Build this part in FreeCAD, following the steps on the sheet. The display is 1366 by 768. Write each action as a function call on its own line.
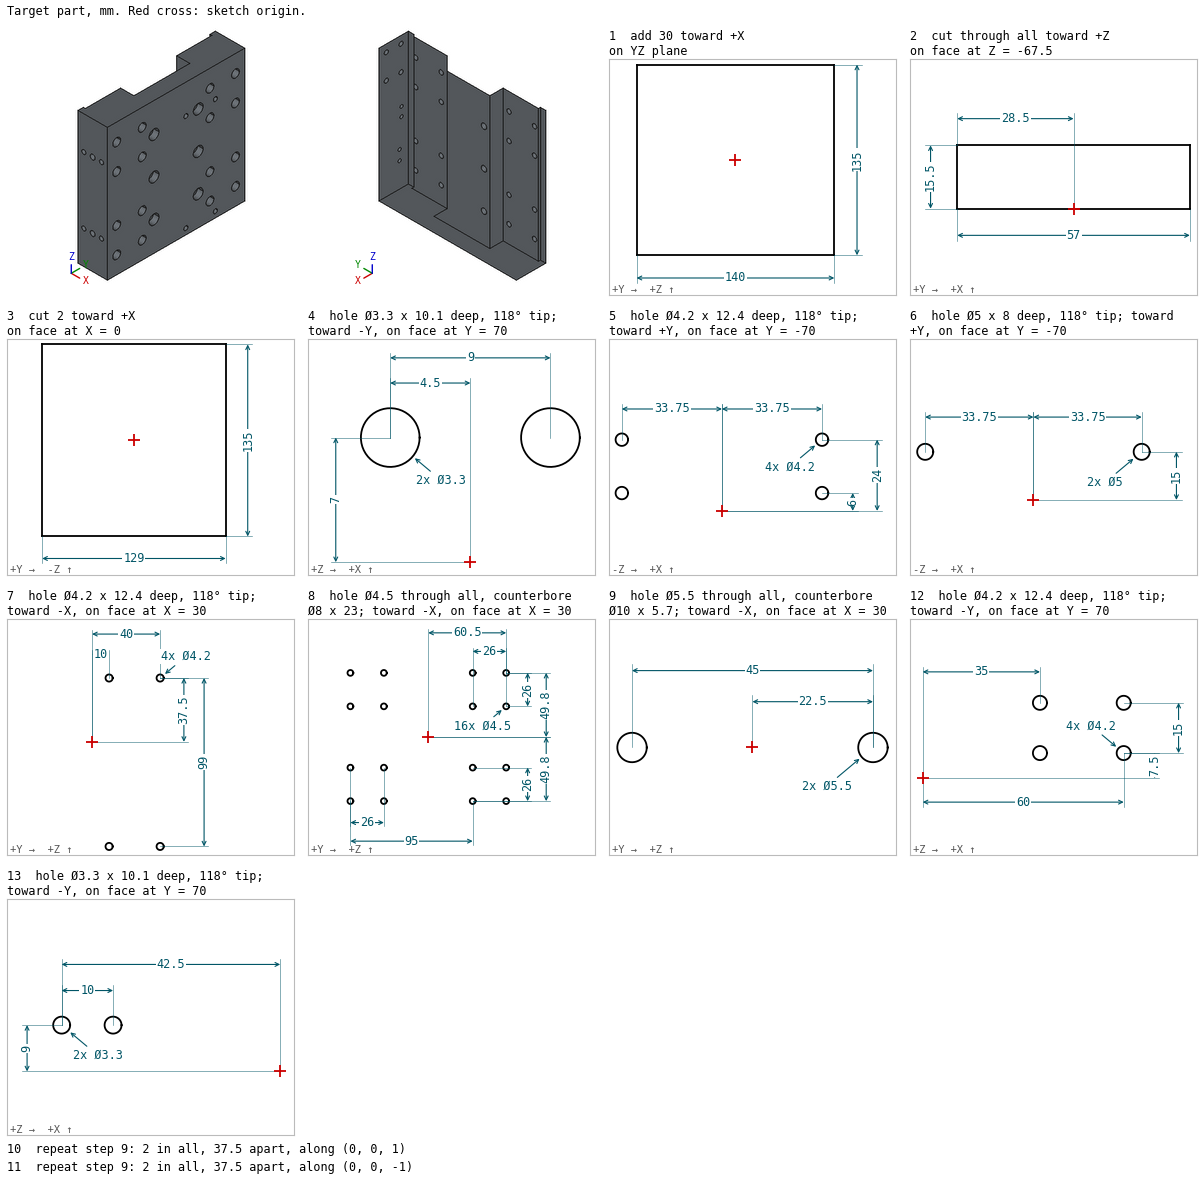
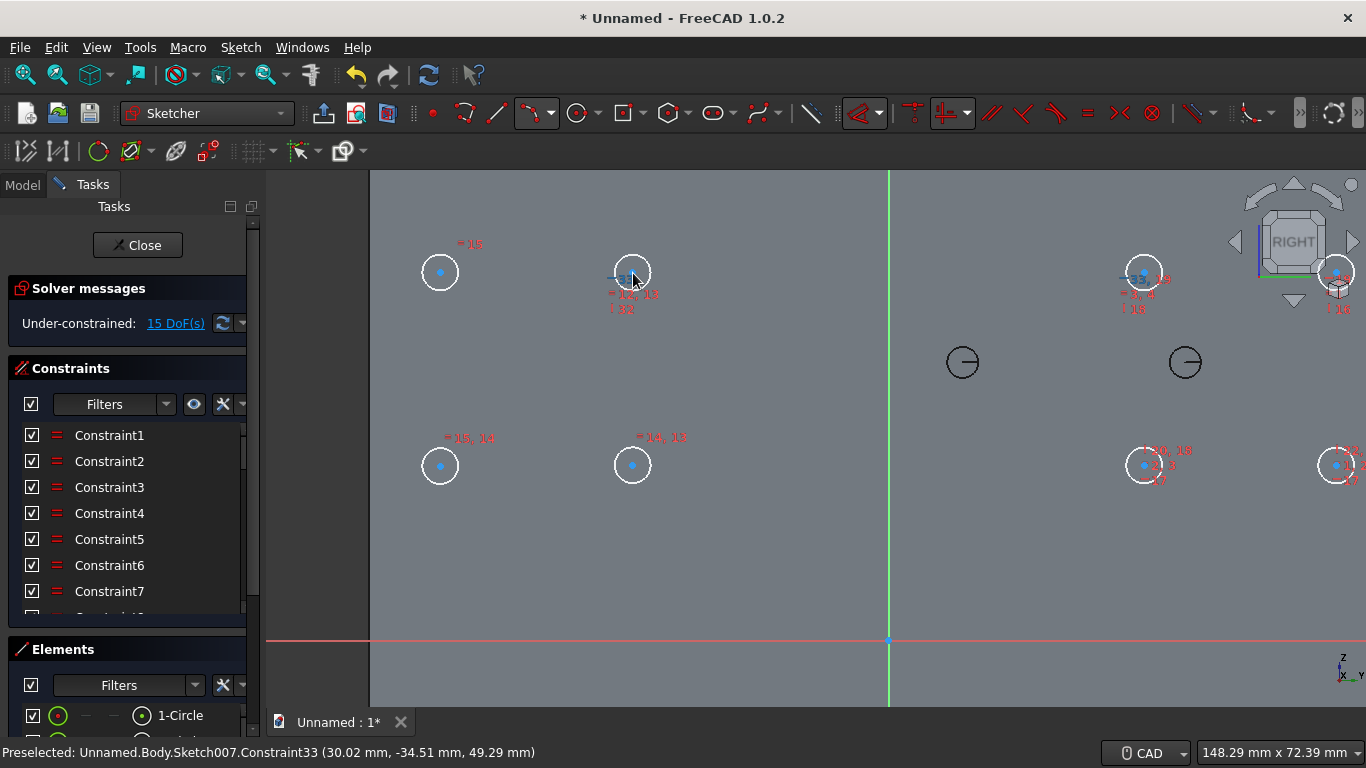
scroll(633, 273, up, 4)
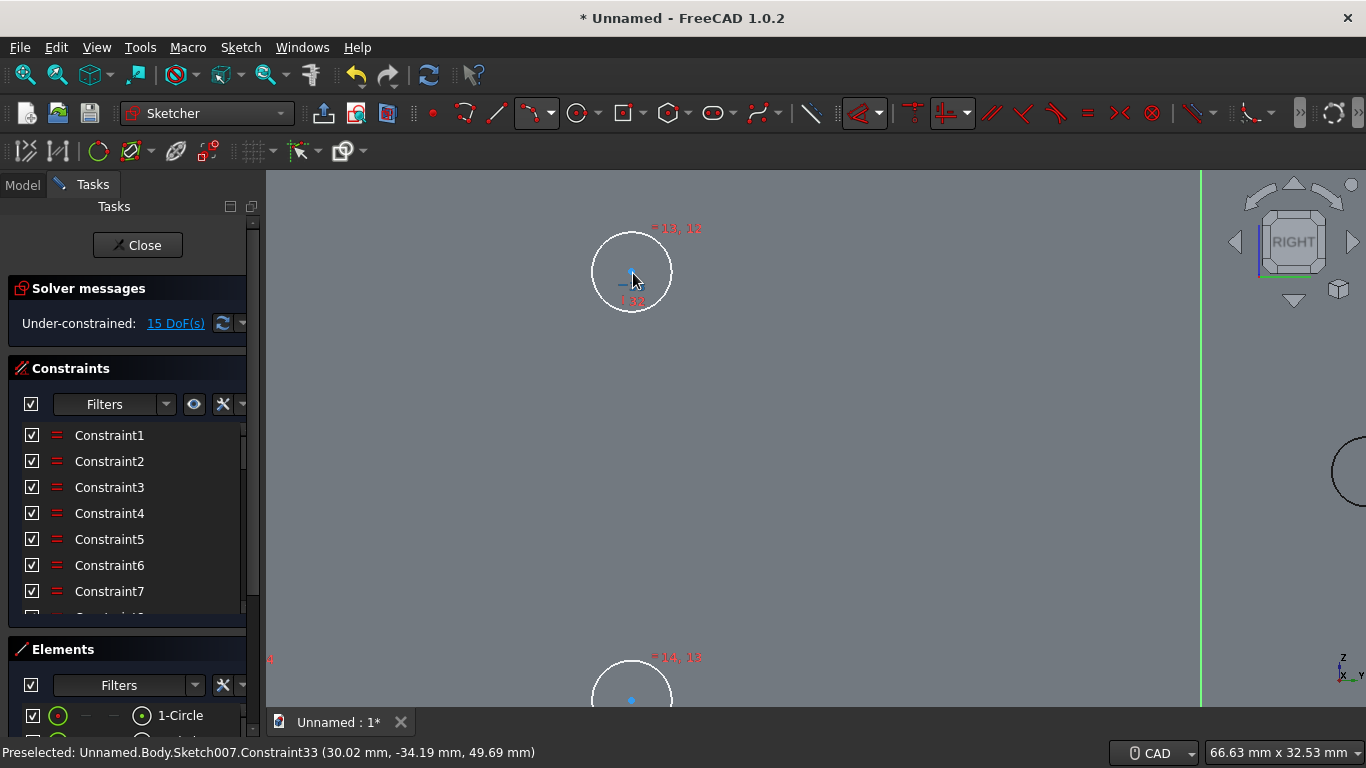
click(632, 272)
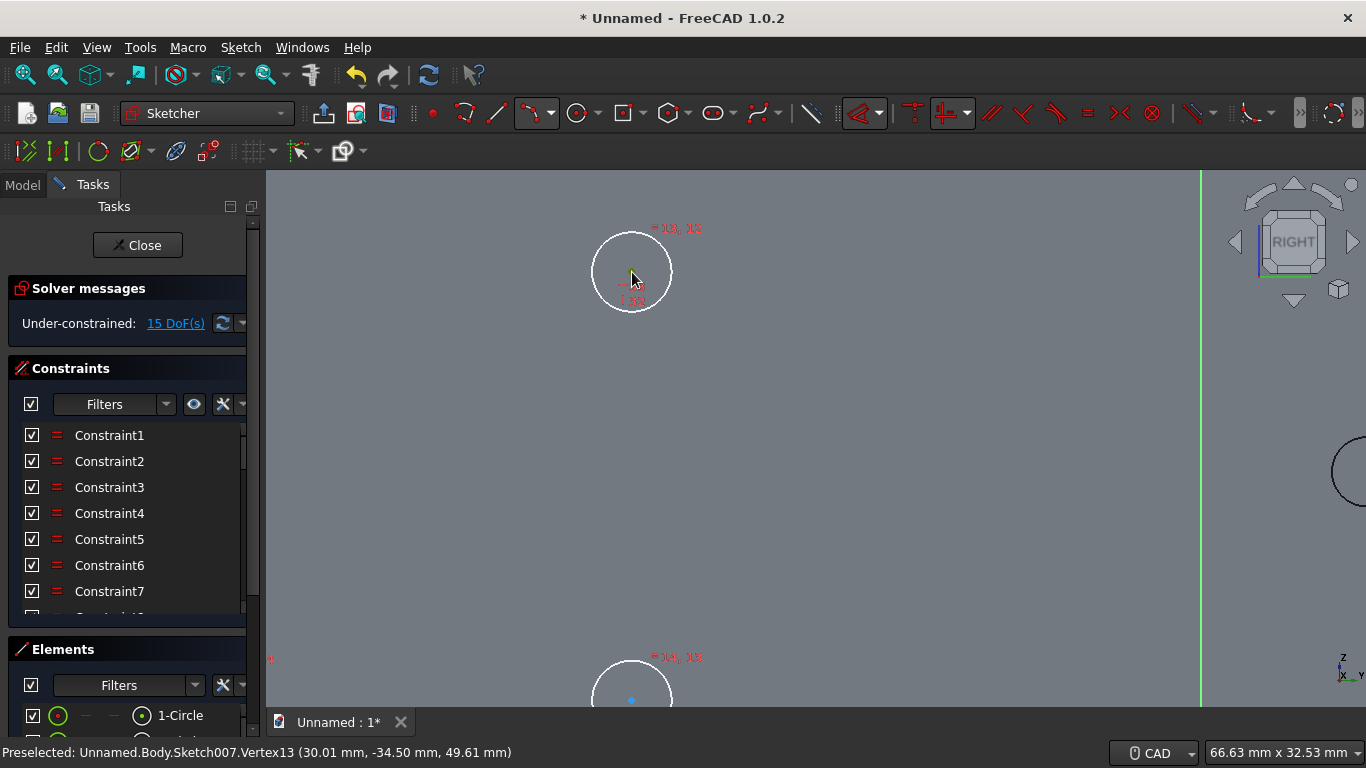
scroll(633, 273, down, 8)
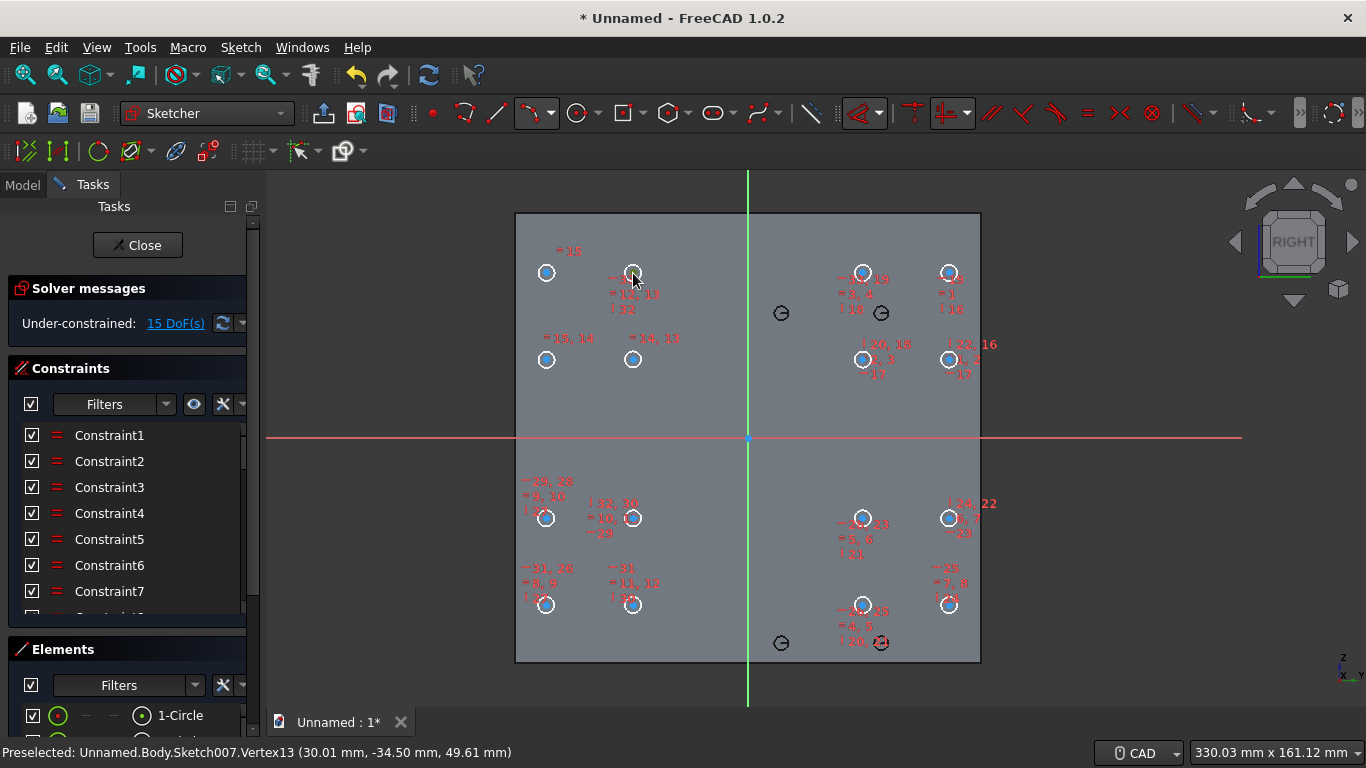
click(633, 359)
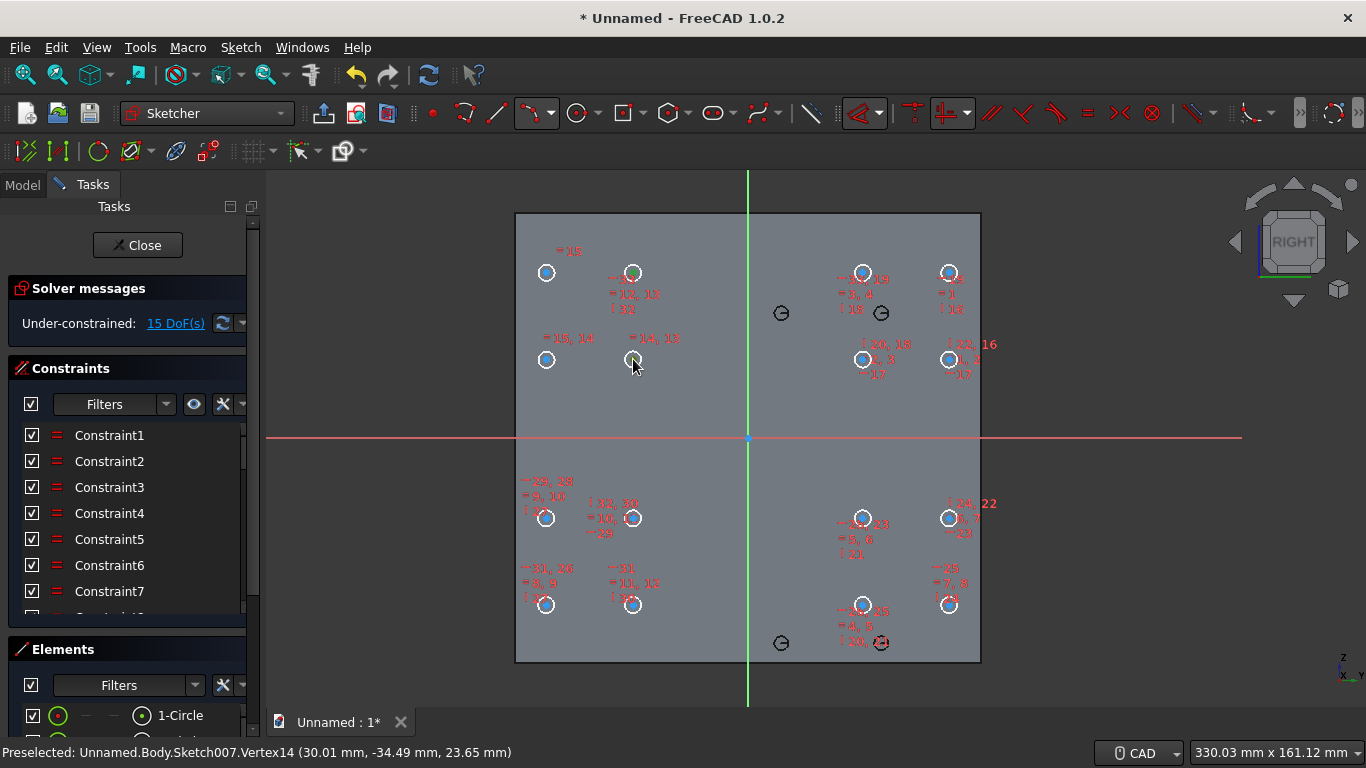
key(v)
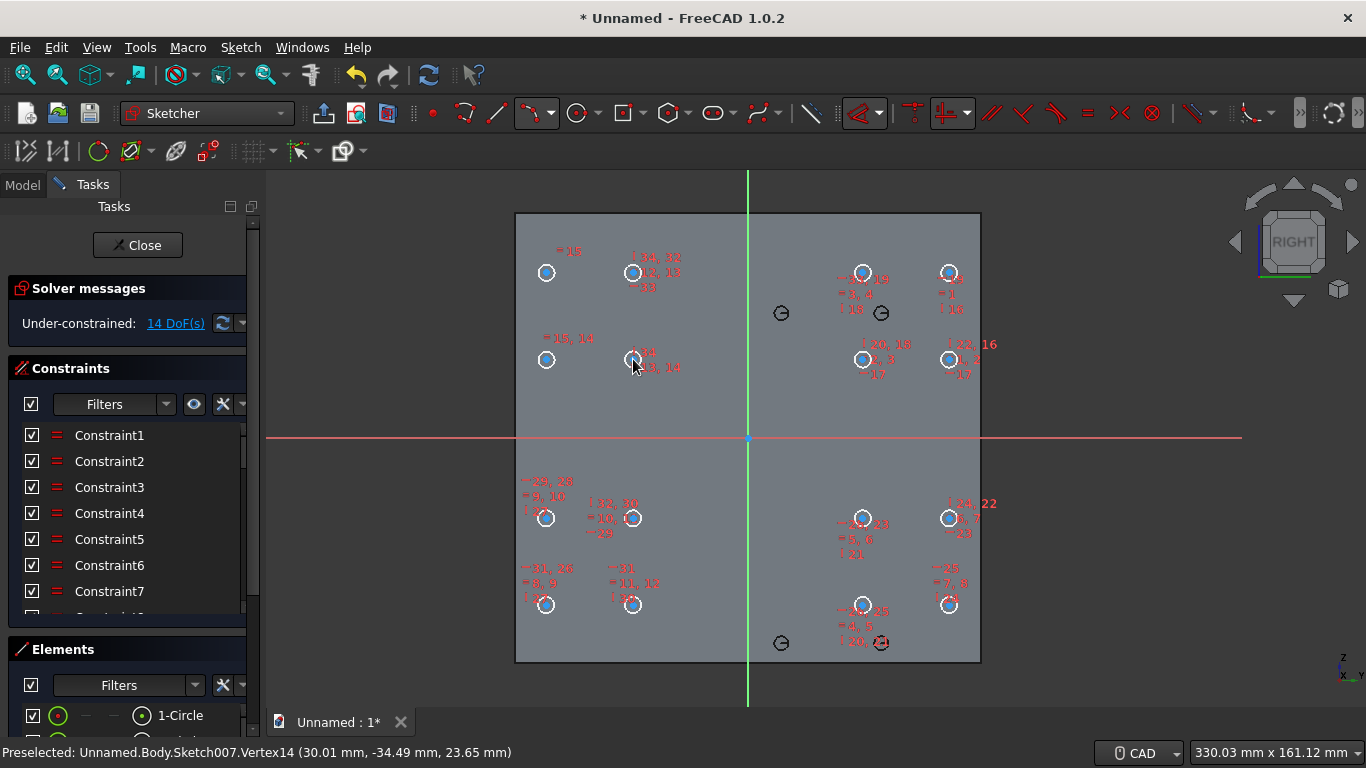
click(863, 360)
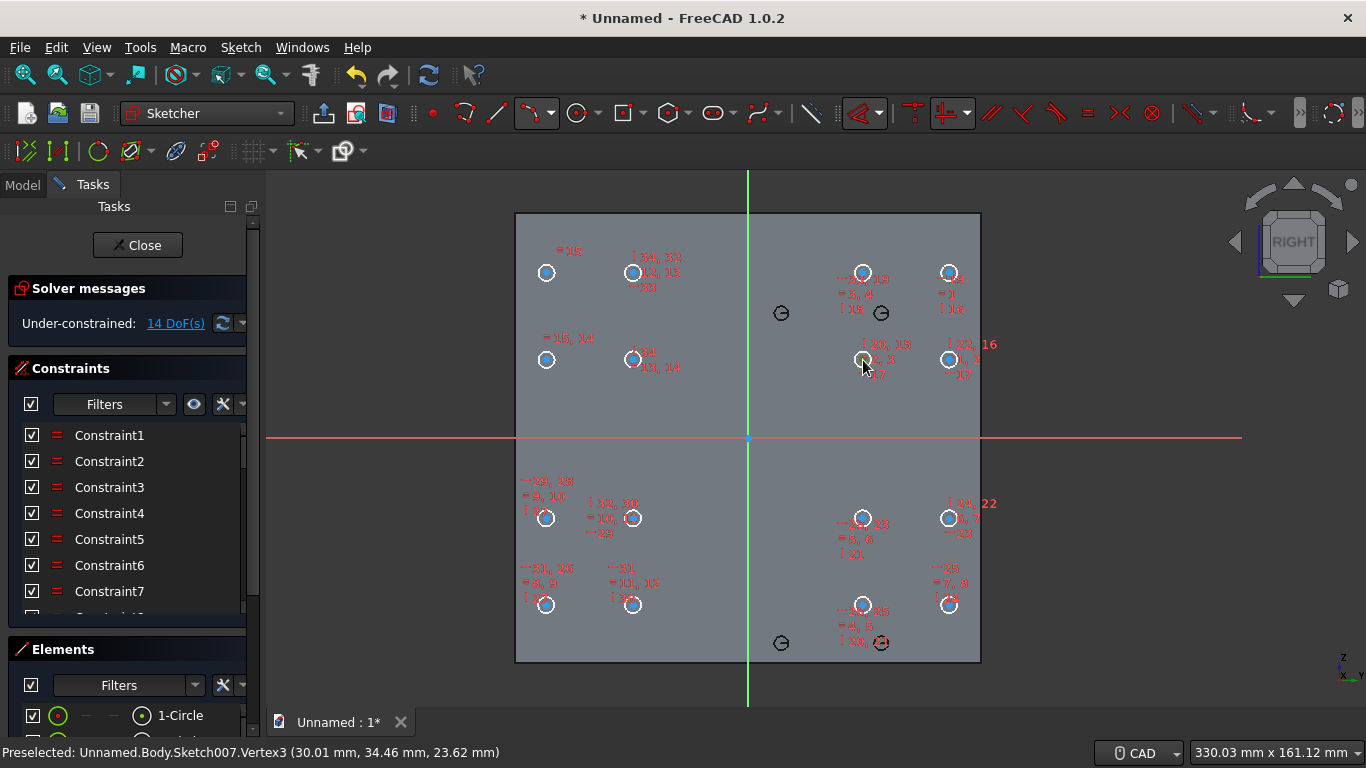
scroll(633, 359, up, 4)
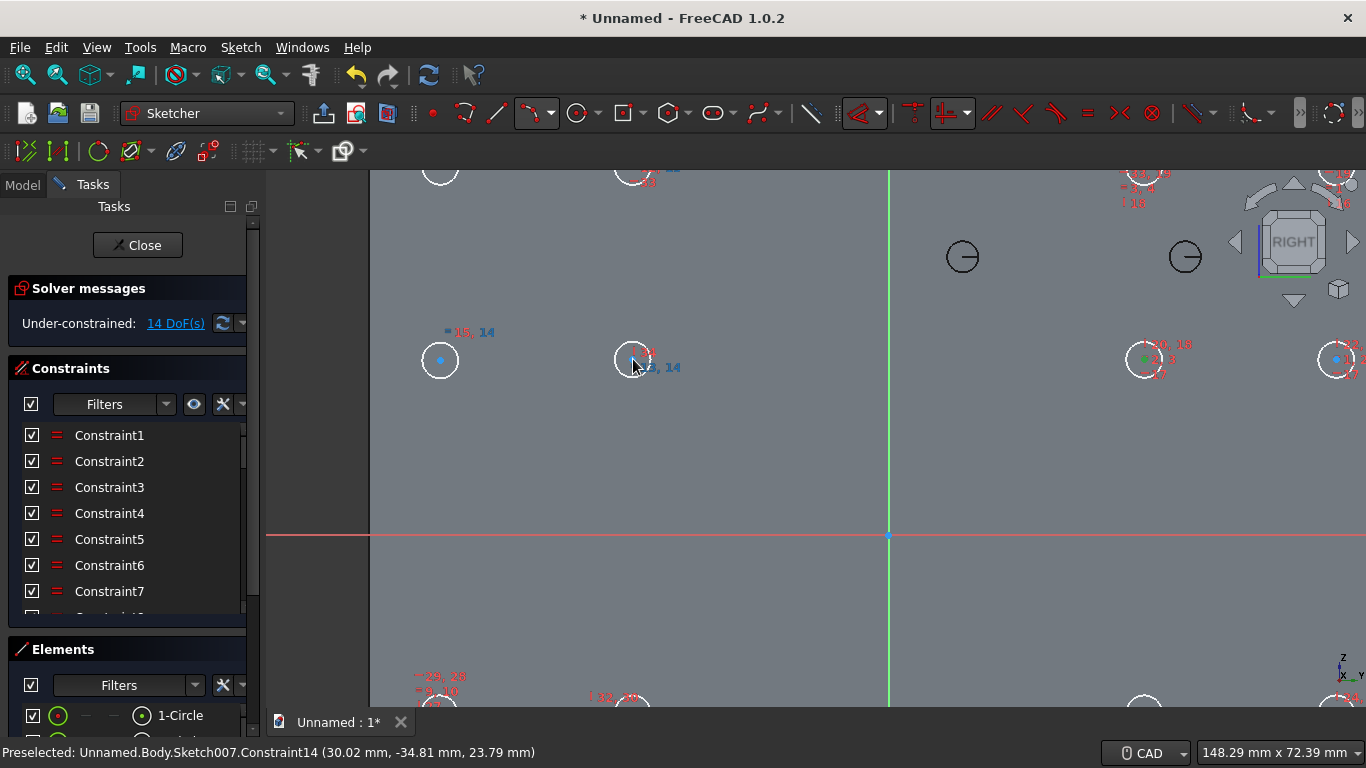
scroll(633, 360, up, 4)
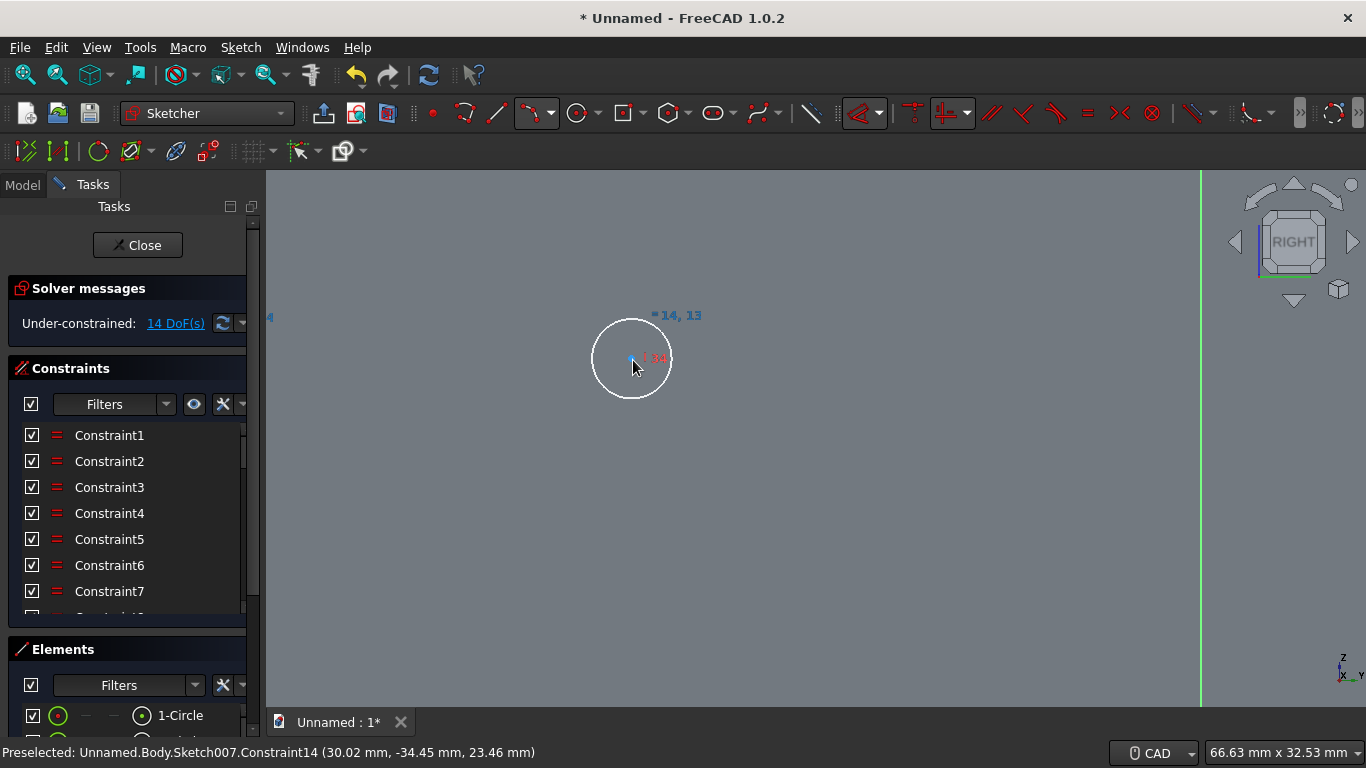
click(632, 359)